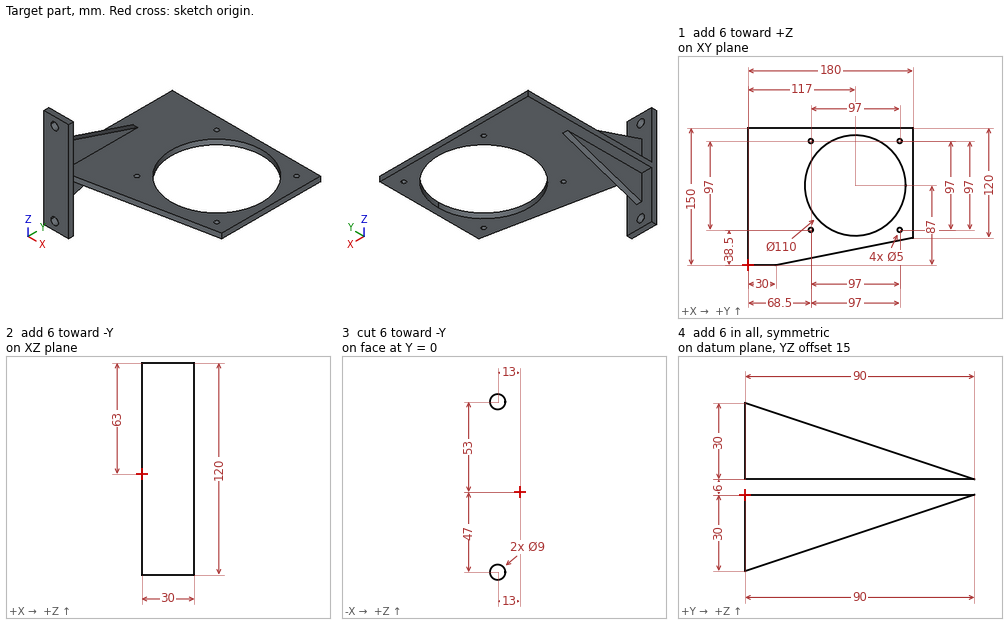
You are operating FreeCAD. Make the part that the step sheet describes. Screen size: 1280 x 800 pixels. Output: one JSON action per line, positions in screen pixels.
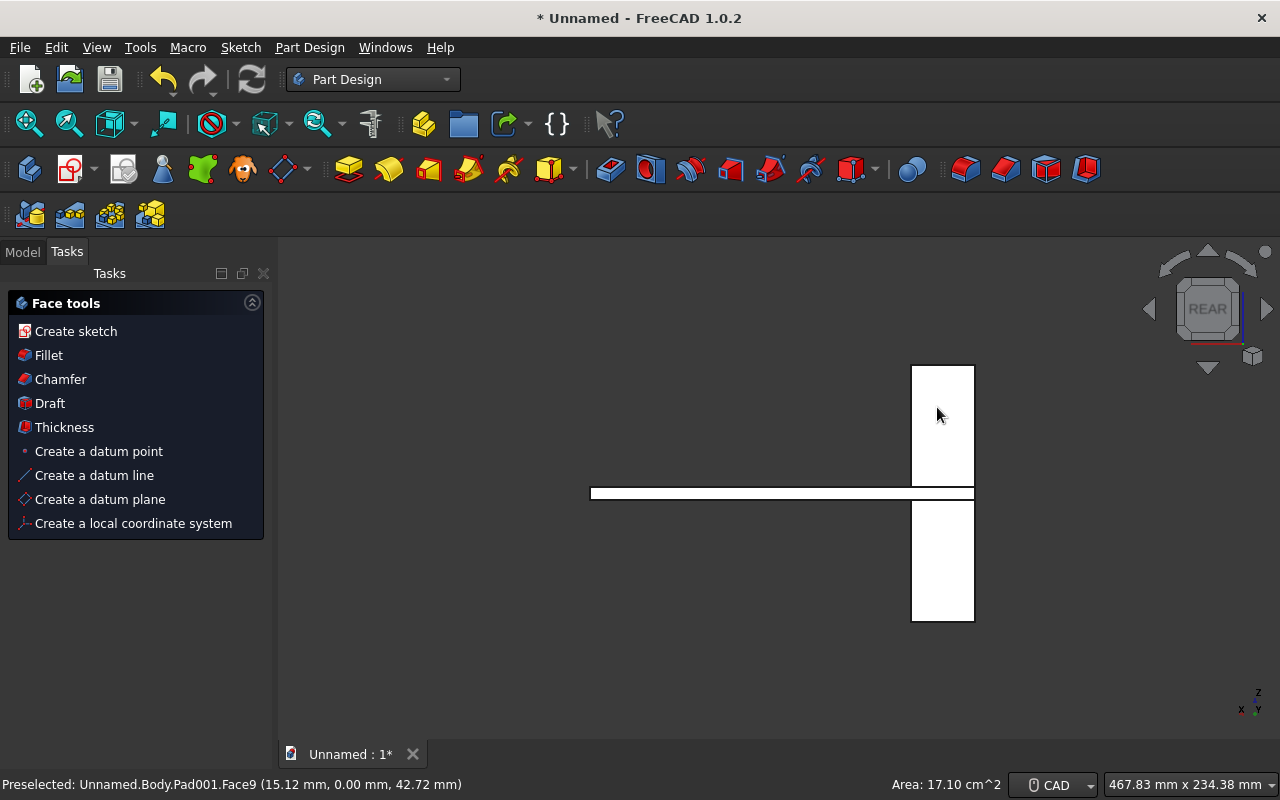
{"action": "left_click", "coordinate": [70, 170]}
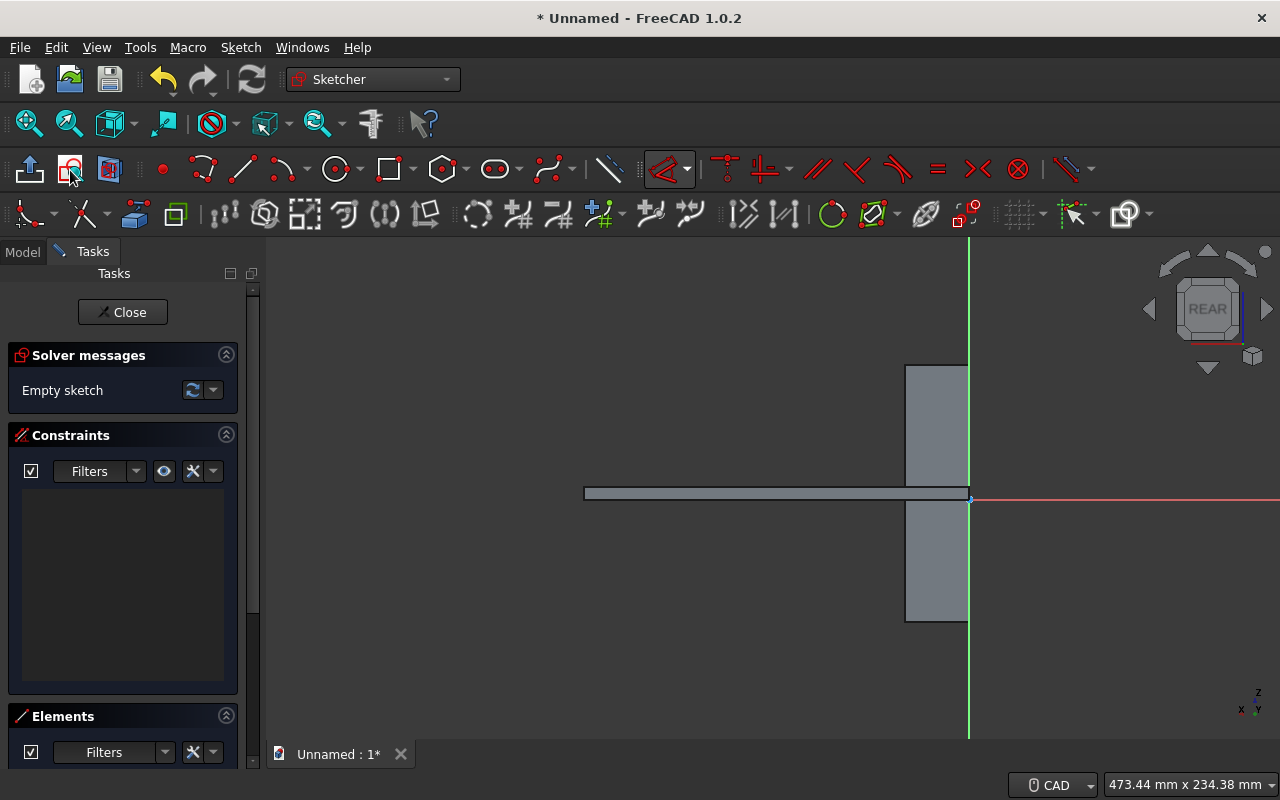
{"action": "key", "text": "q s"}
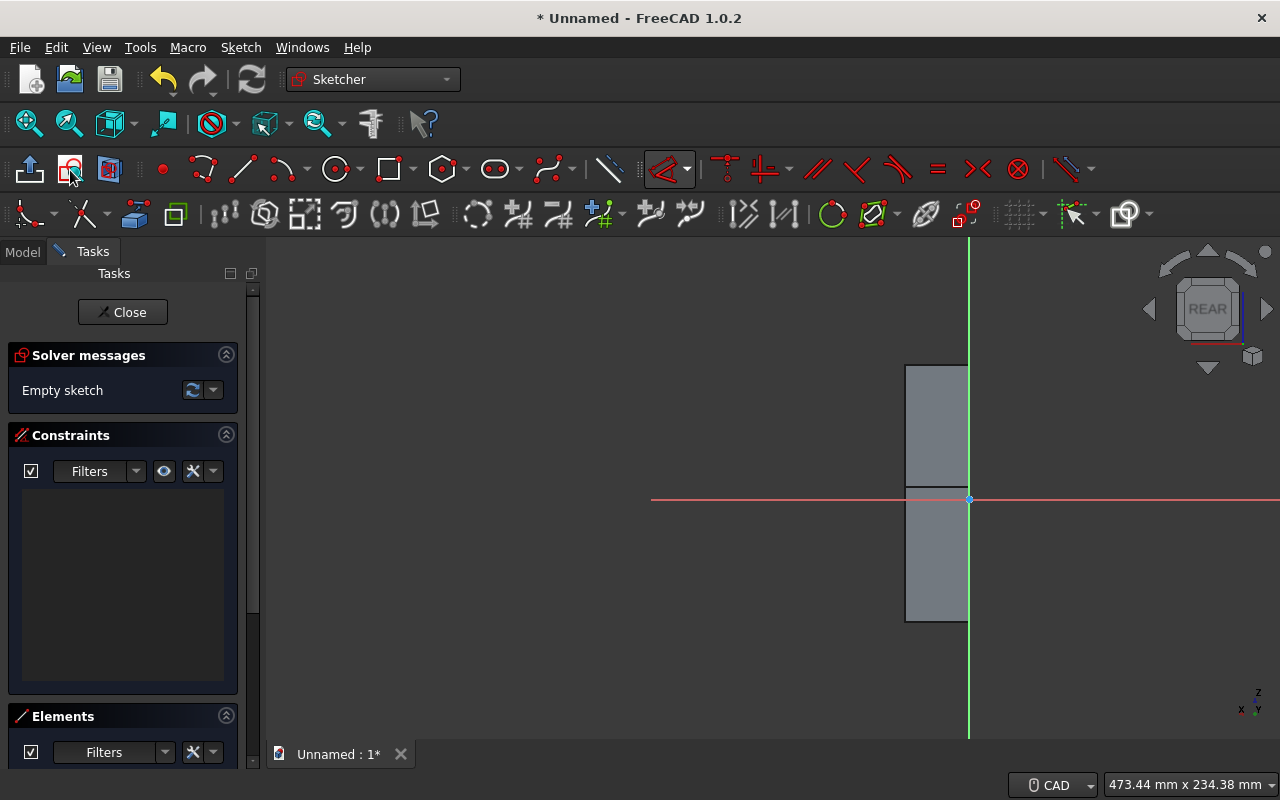
{"action": "key", "text": "g c"}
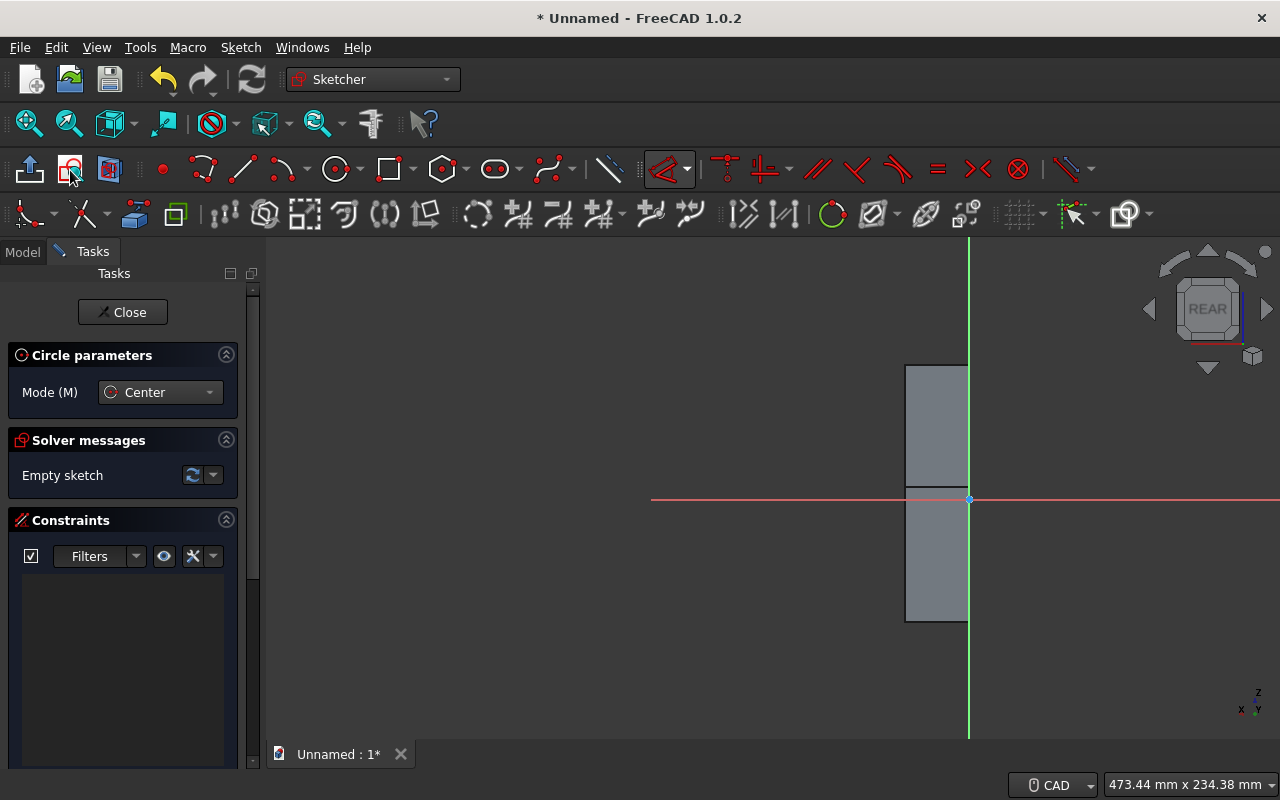
{"action": "scroll", "coordinate": [942, 600], "scroll_direction": "up", "scroll_amount": 5}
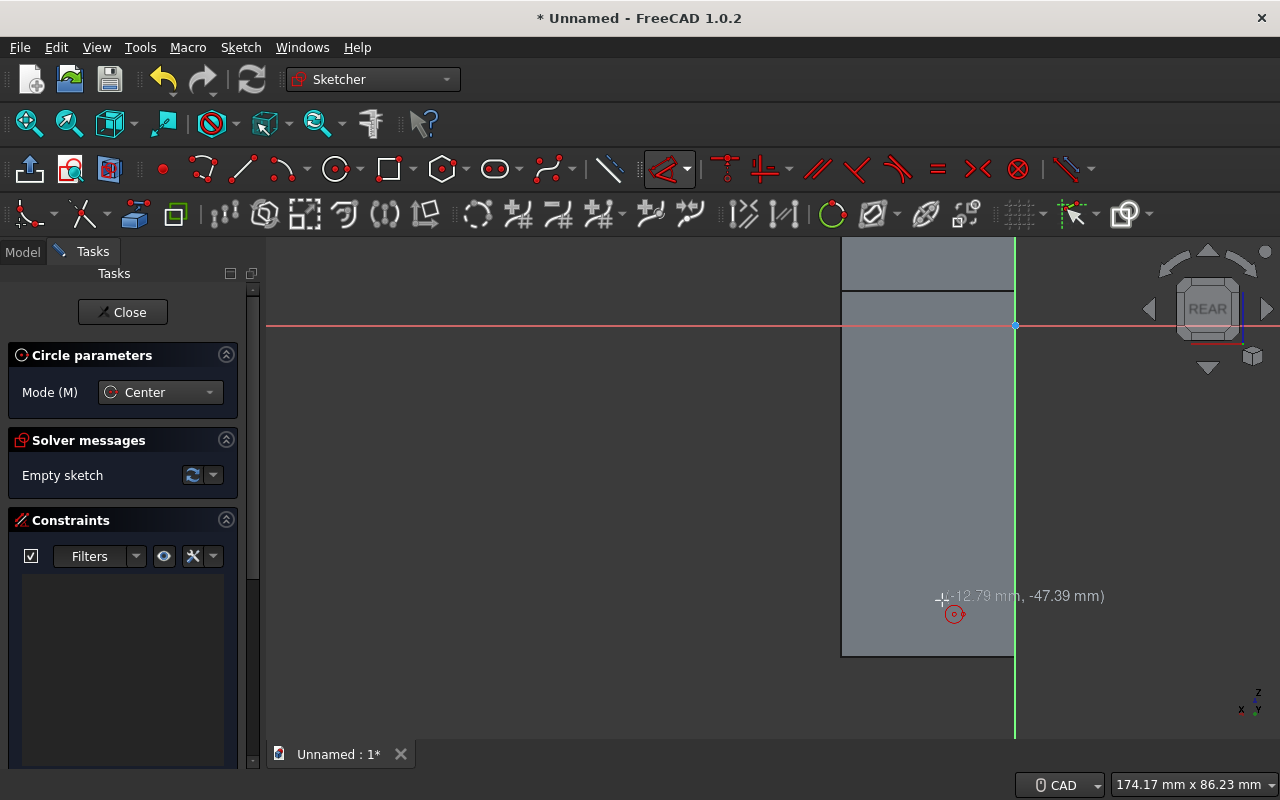
{"action": "left_click", "coordinate": [940, 599]}
{"action": "mouse_move", "coordinate": [958, 581]}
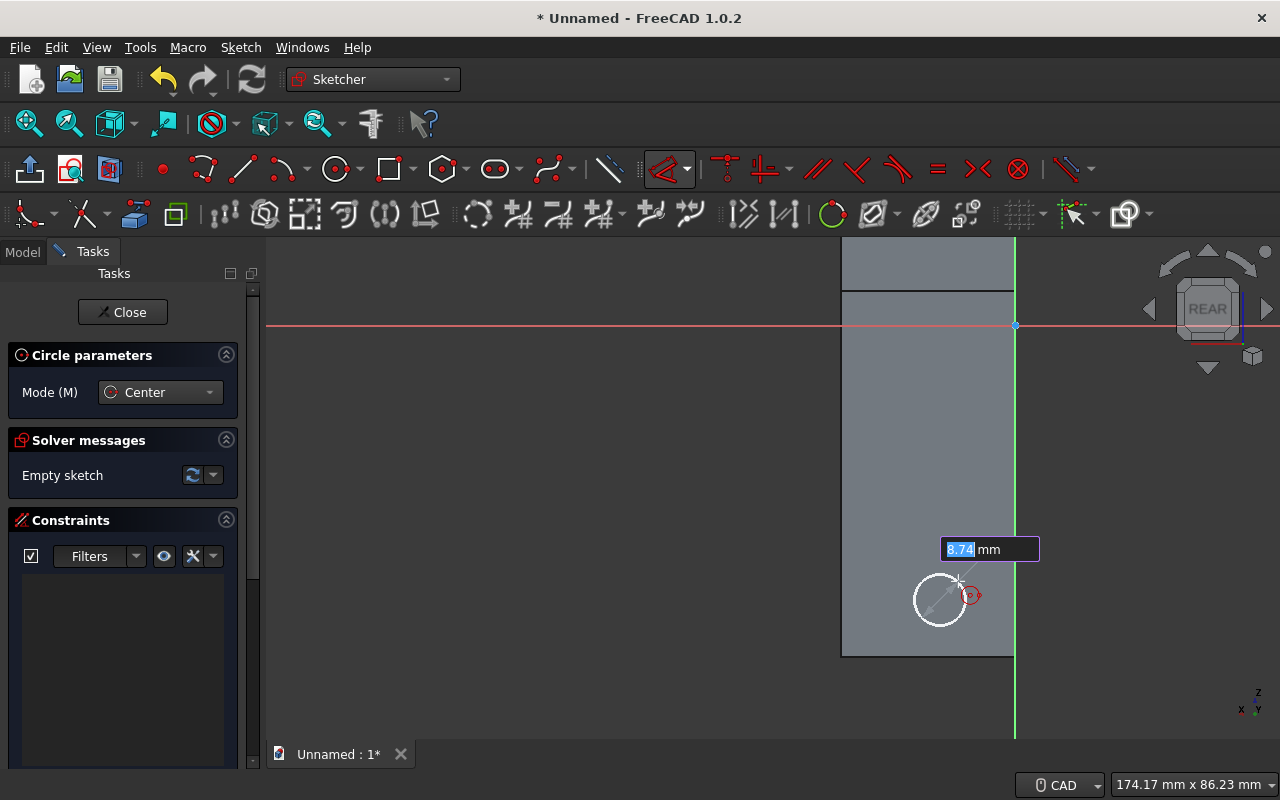
{"action": "type", "text": "9"}
{"action": "key", "text": "Return"}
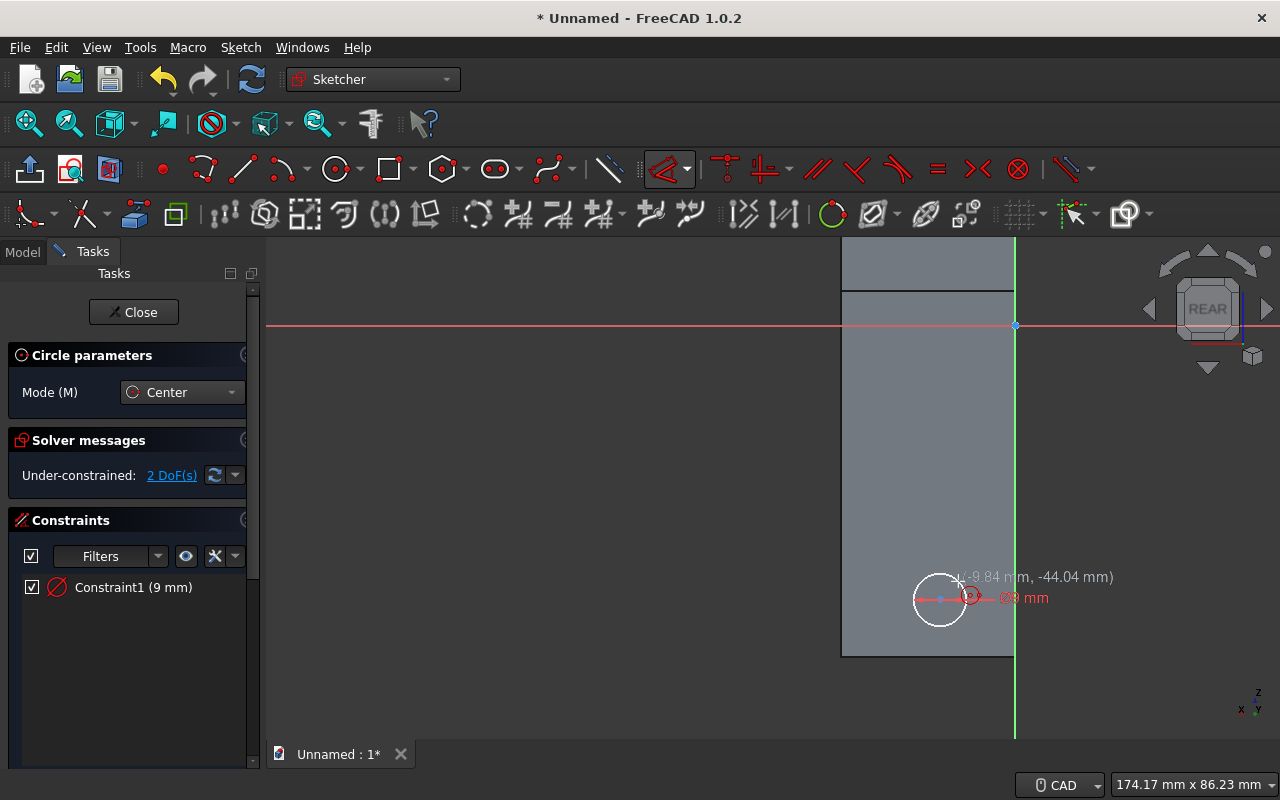
{"action": "scroll", "coordinate": [492, 635], "scroll_direction": "down", "scroll_amount": 4}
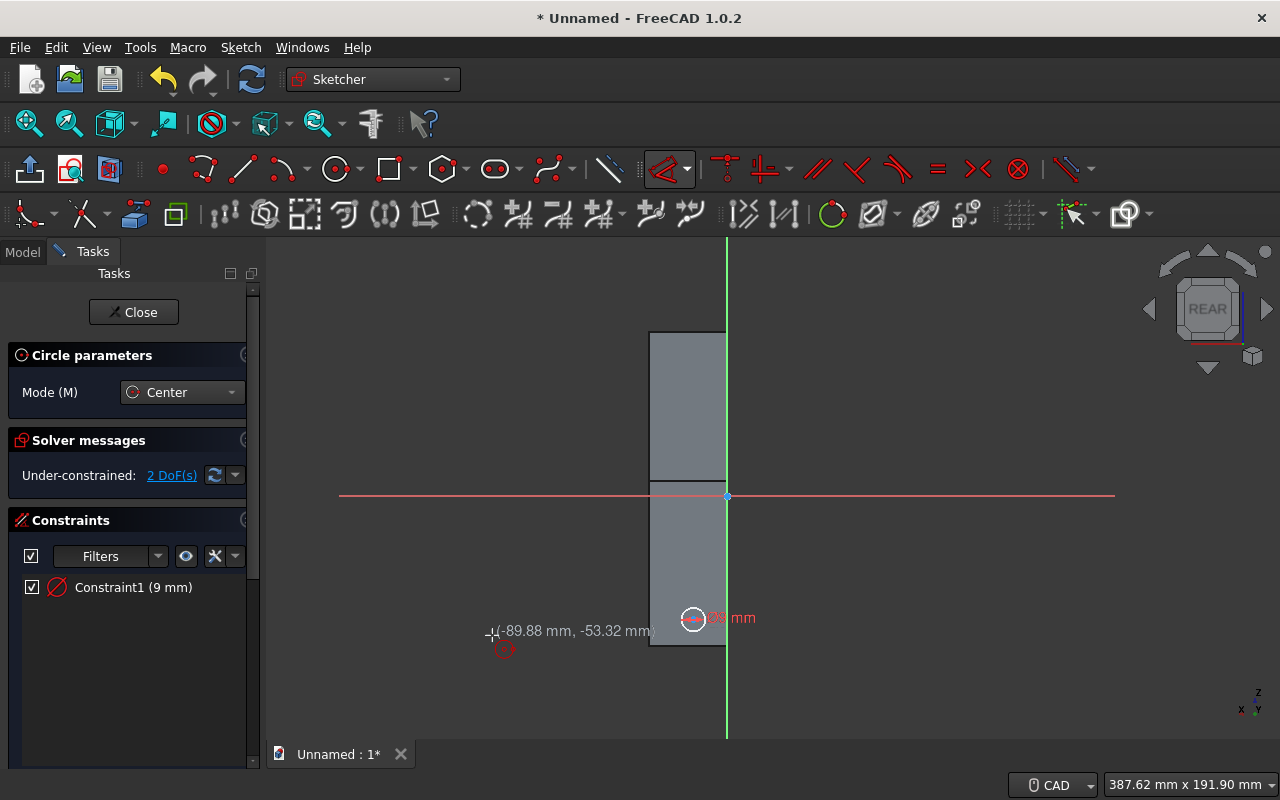
{"action": "scroll", "coordinate": [693, 358], "scroll_direction": "up", "scroll_amount": 4}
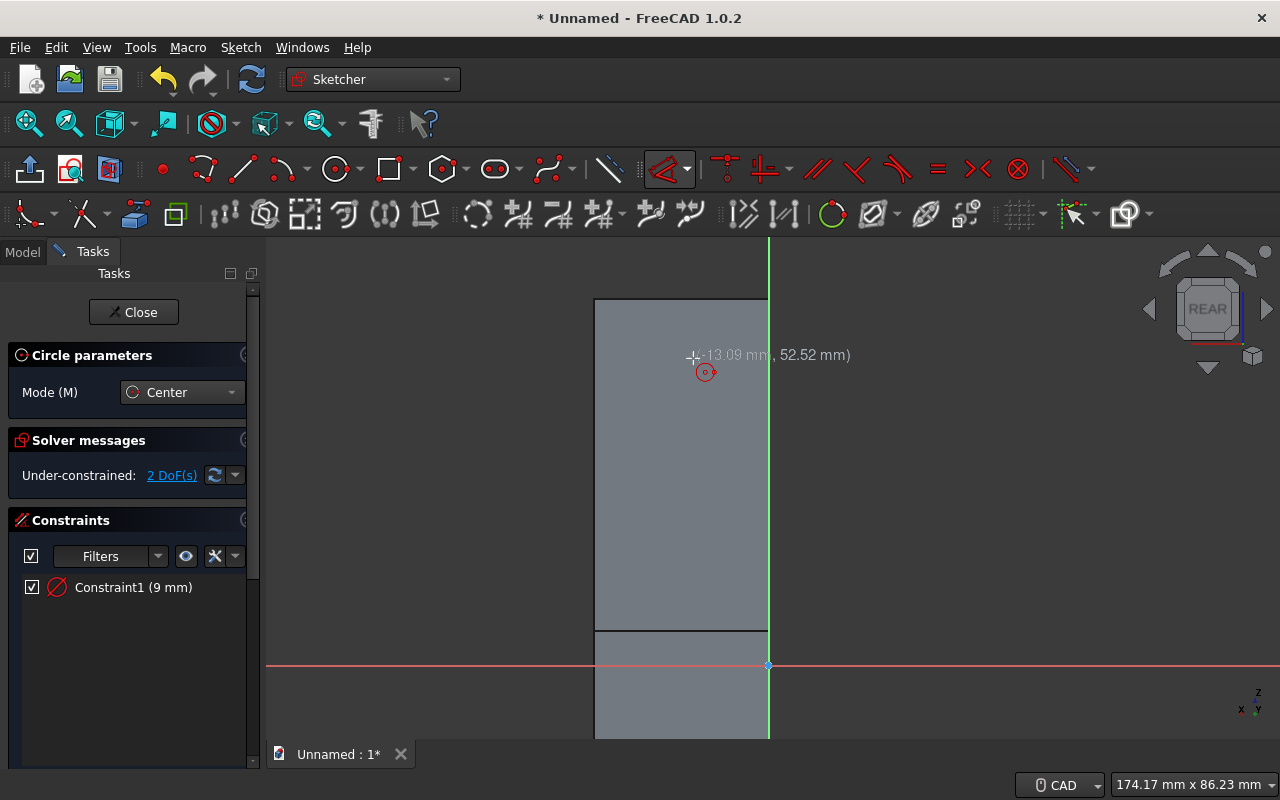
{"action": "left_click", "coordinate": [693, 357]}
{"action": "mouse_move", "coordinate": [712, 339]}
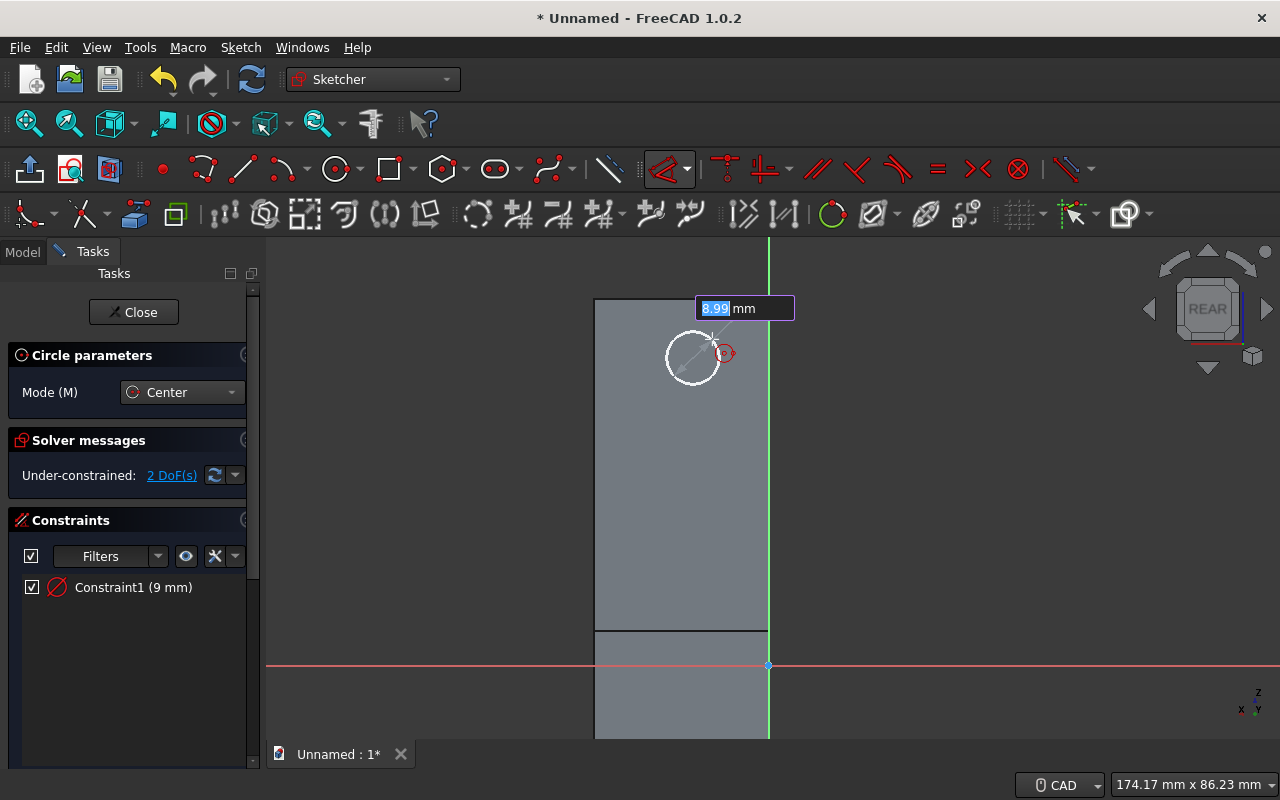
{"action": "type", "text": "9"}
{"action": "key", "text": "Return"}
{"action": "key", "text": "Escape"}